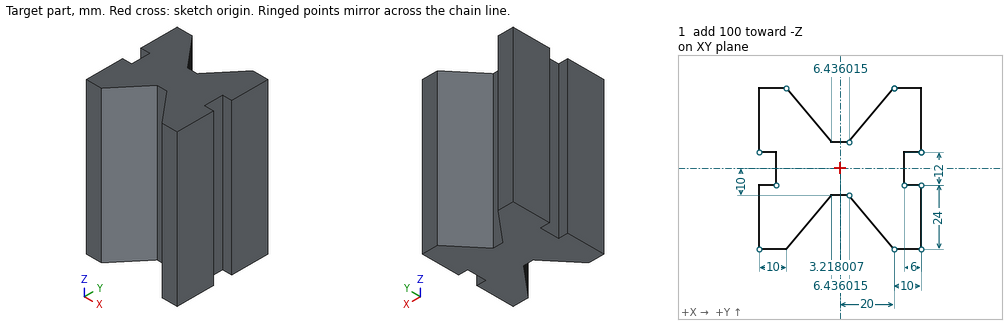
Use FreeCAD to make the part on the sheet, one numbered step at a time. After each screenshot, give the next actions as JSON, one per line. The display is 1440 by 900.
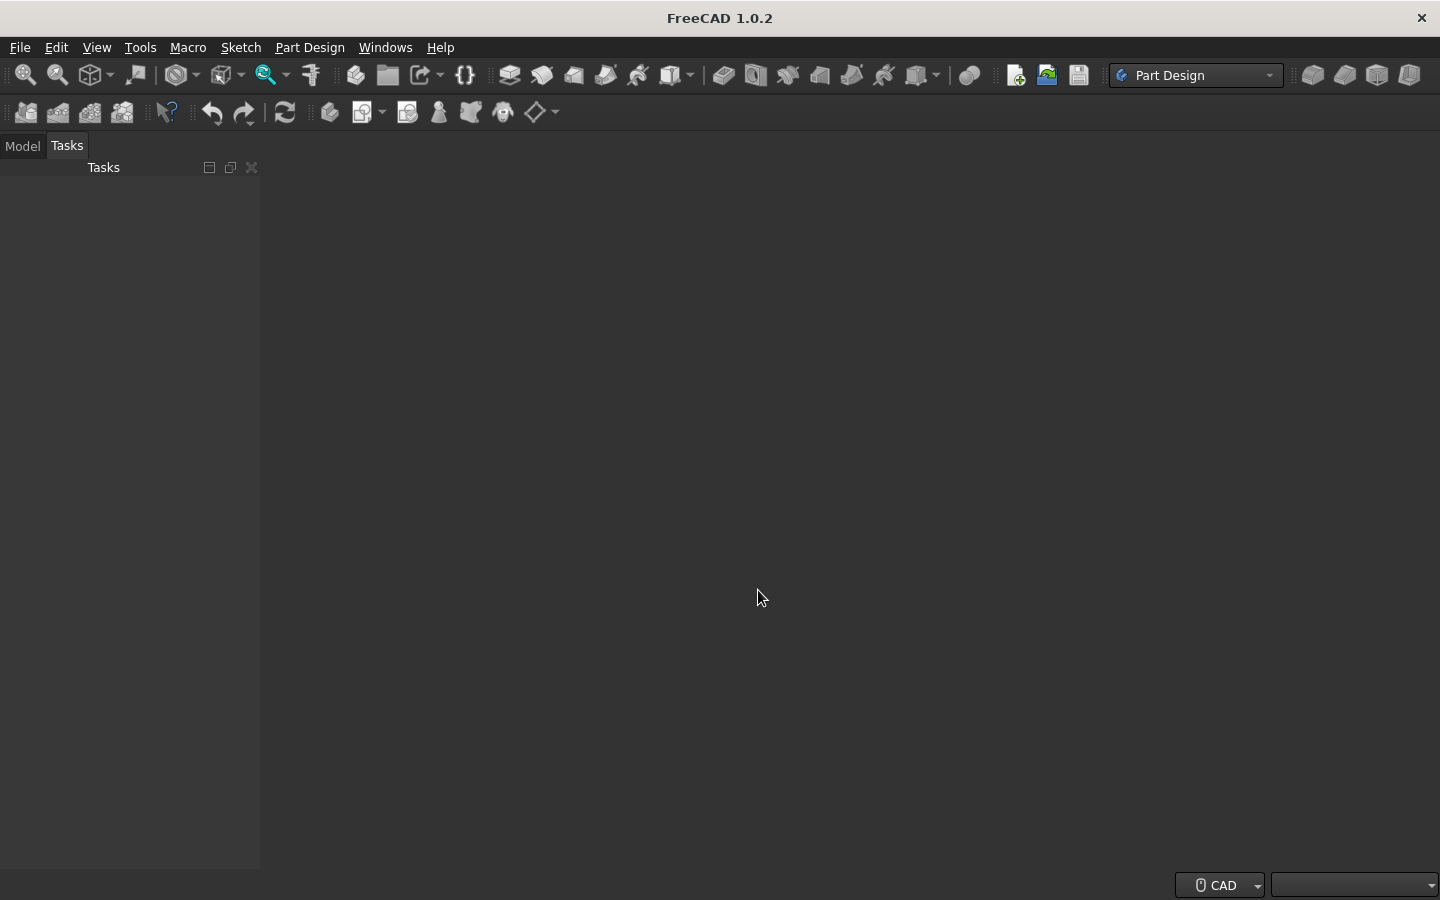
{"action": "key", "text": "ctrl+n"}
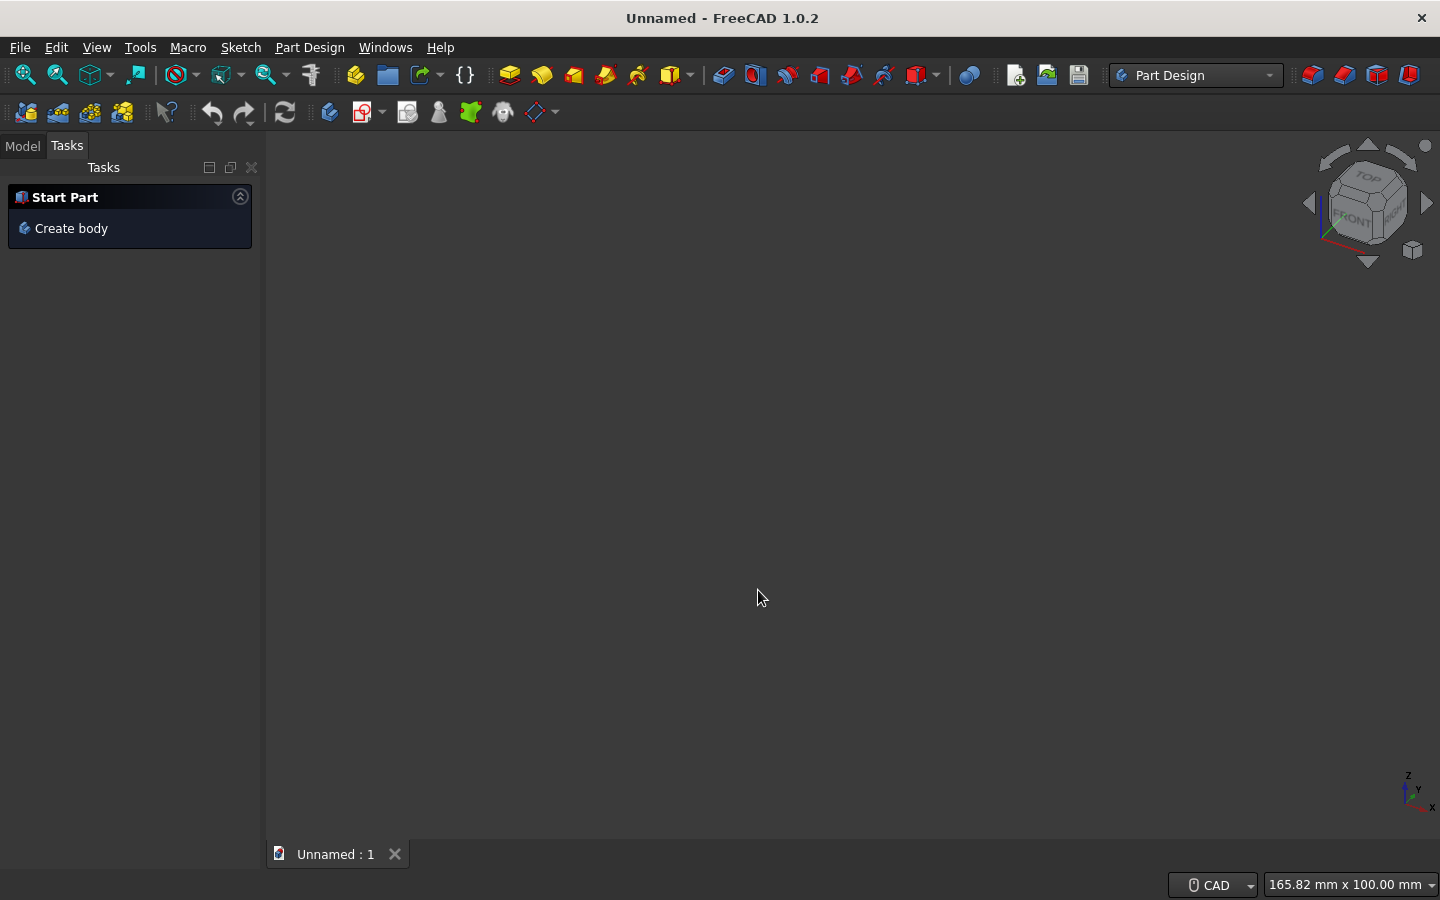
{"action": "left_click", "coordinate": [362, 112]}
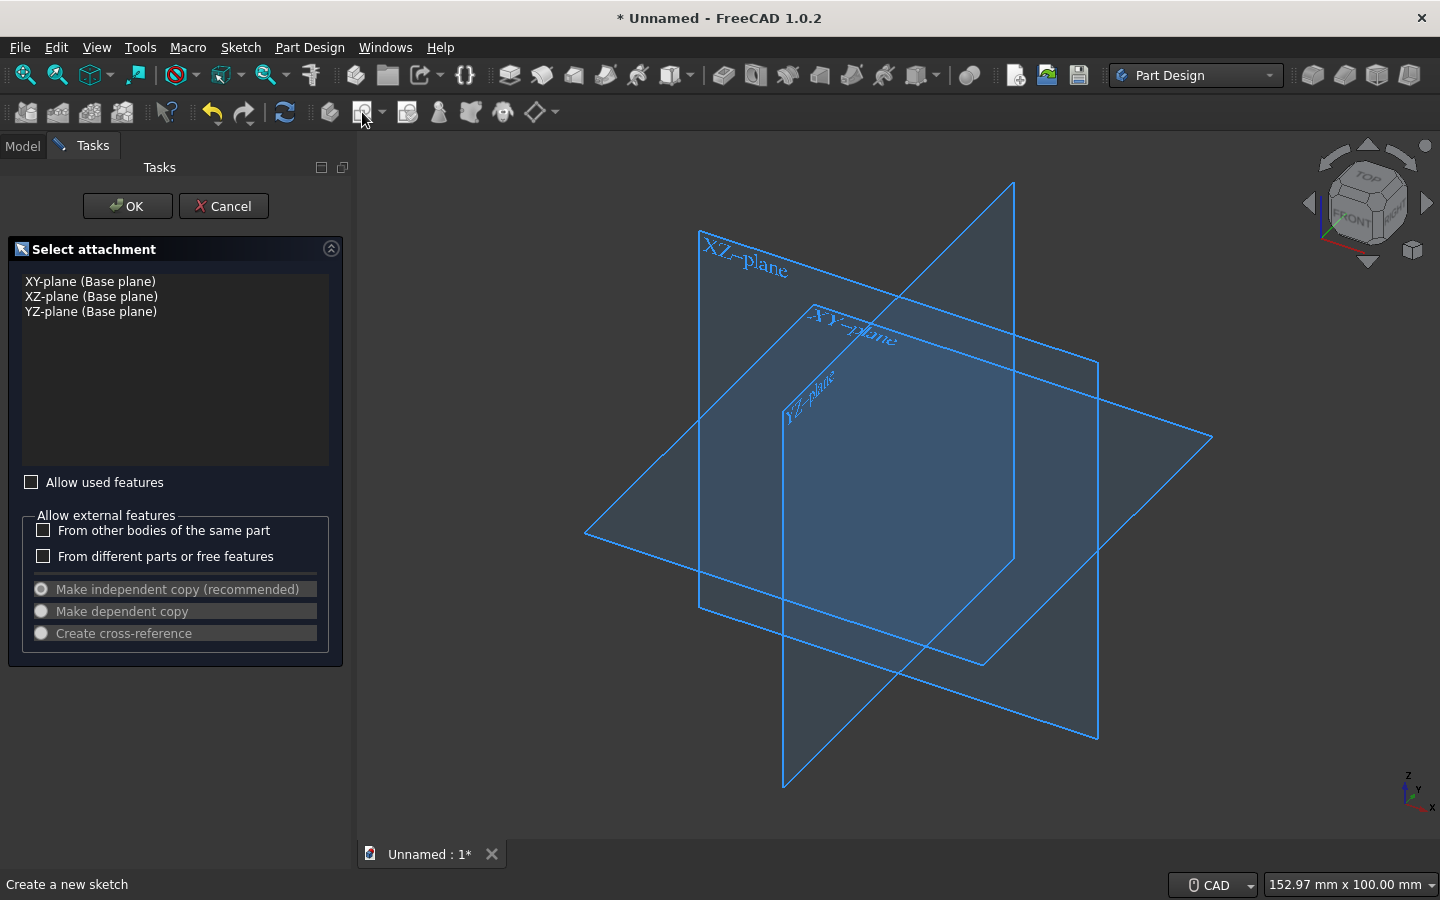
{"action": "left_click", "coordinate": [82, 282]}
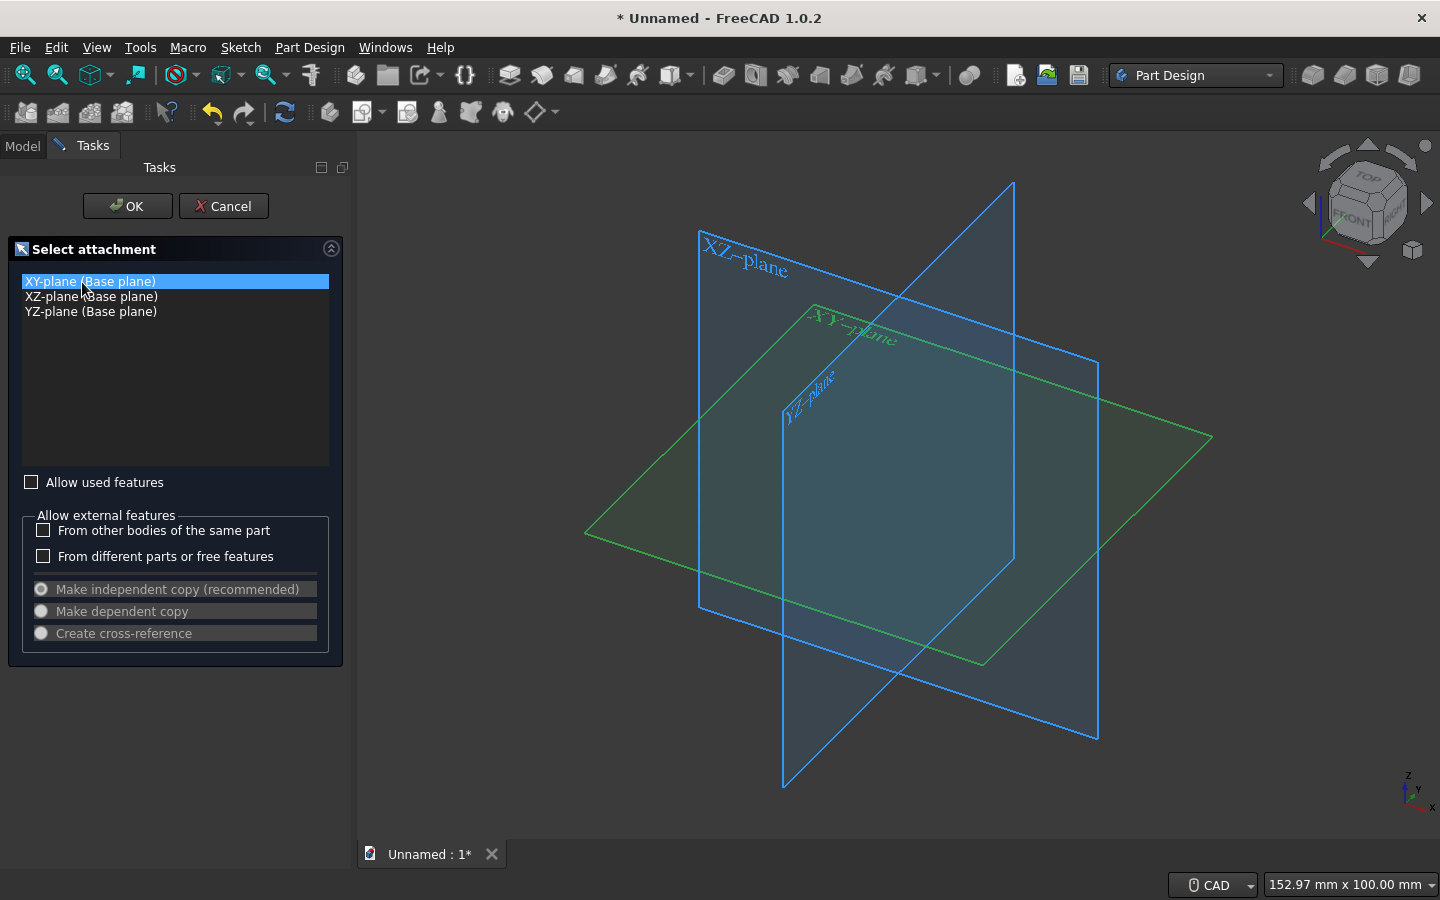
{"action": "left_click", "coordinate": [128, 206]}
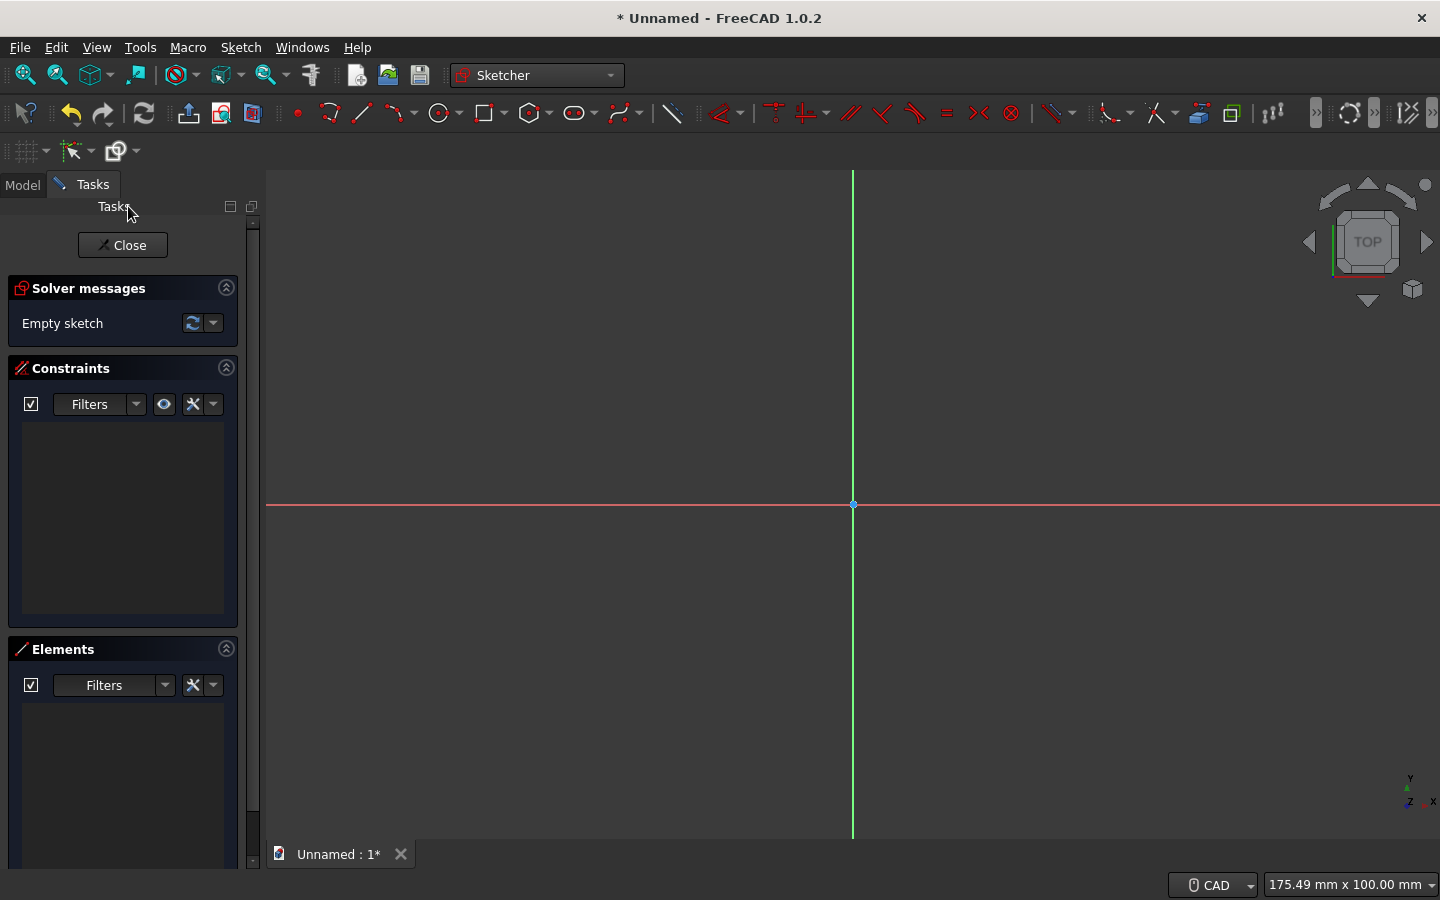
{"action": "key", "text": "g m"}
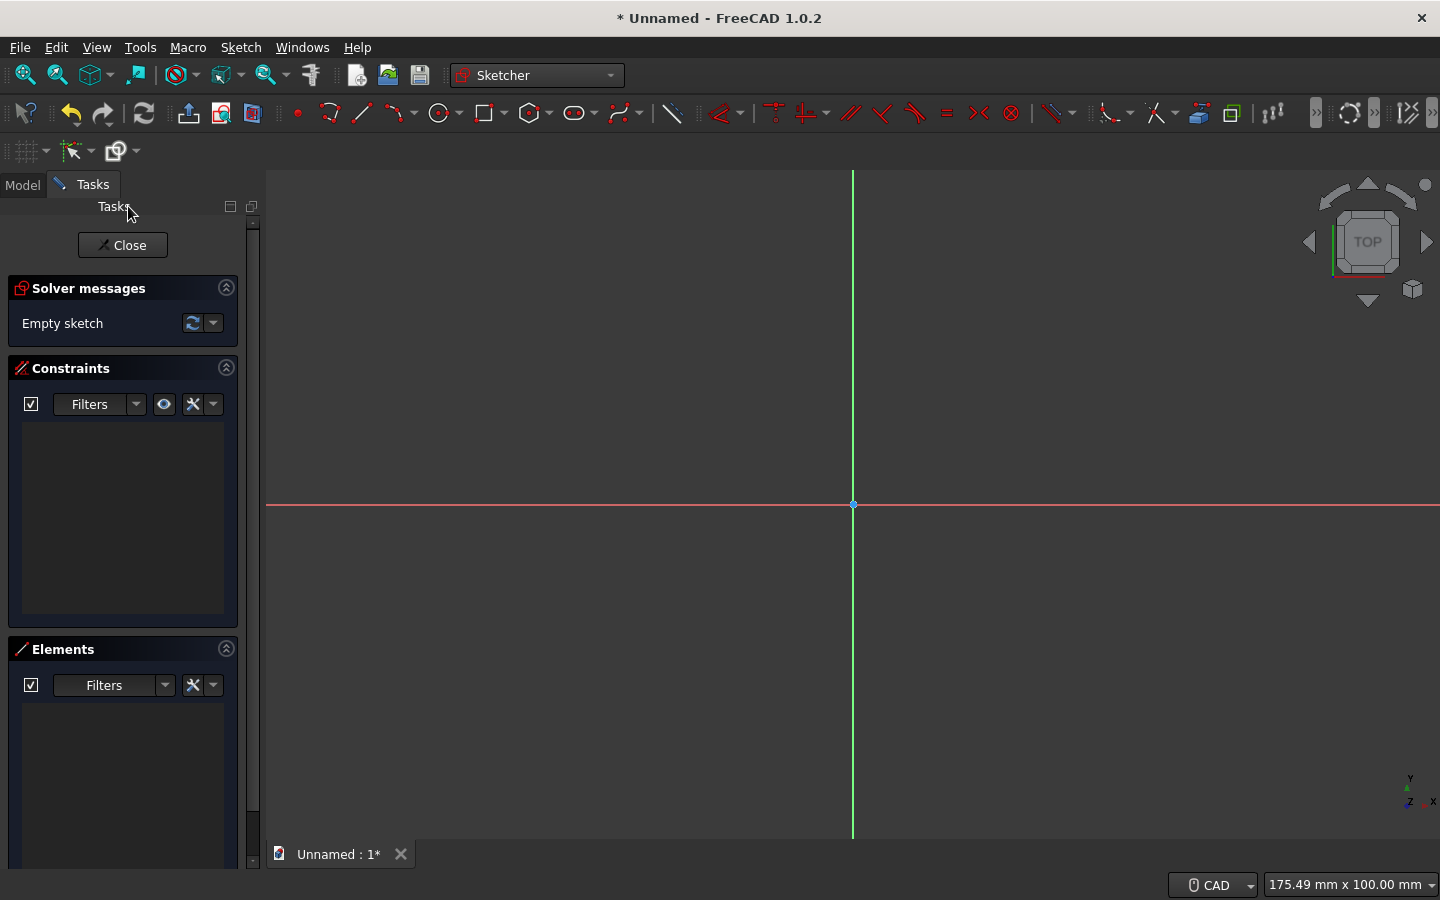
{"action": "left_click", "coordinate": [831, 571]}
{"action": "left_click", "coordinate": [875, 571]}
{"action": "left_click", "coordinate": [987, 705]}
{"action": "left_click", "coordinate": [1054, 705]}
{"action": "left_click", "coordinate": [1054, 545]}
{"action": "left_click", "coordinate": [1014, 545]}
{"action": "left_click", "coordinate": [1014, 464]}
{"action": "left_click", "coordinate": [1054, 464]}
{"action": "left_click", "coordinate": [1054, 304]}
{"action": "left_click", "coordinate": [987, 304]}
{"action": "left_click", "coordinate": [875, 438]}
{"action": "left_click", "coordinate": [831, 438]}
{"action": "left_click", "coordinate": [719, 304]}
{"action": "left_click", "coordinate": [652, 304]}
{"action": "left_click", "coordinate": [652, 464]}
{"action": "left_click", "coordinate": [692, 464]}
{"action": "left_click", "coordinate": [692, 545]}
{"action": "left_click", "coordinate": [652, 545]}
{"action": "left_click", "coordinate": [652, 705]}
{"action": "left_click", "coordinate": [719, 705]}
{"action": "left_click", "coordinate": [831, 572]}
{"action": "key", "text": "Escape"}
{"action": "key", "text": "Escape"}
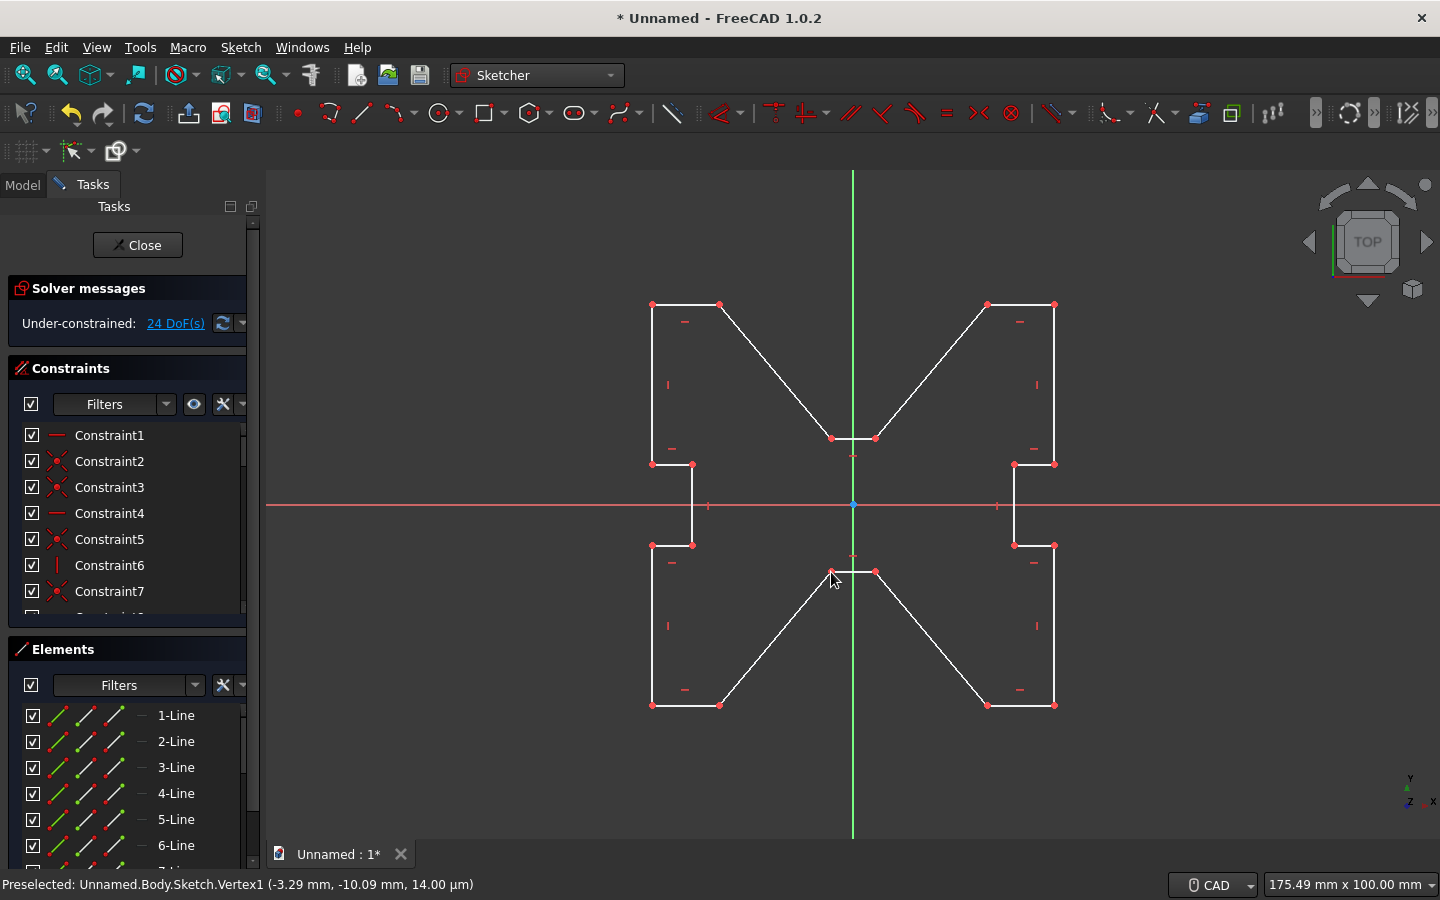
{"action": "left_click", "coordinate": [1054, 546]}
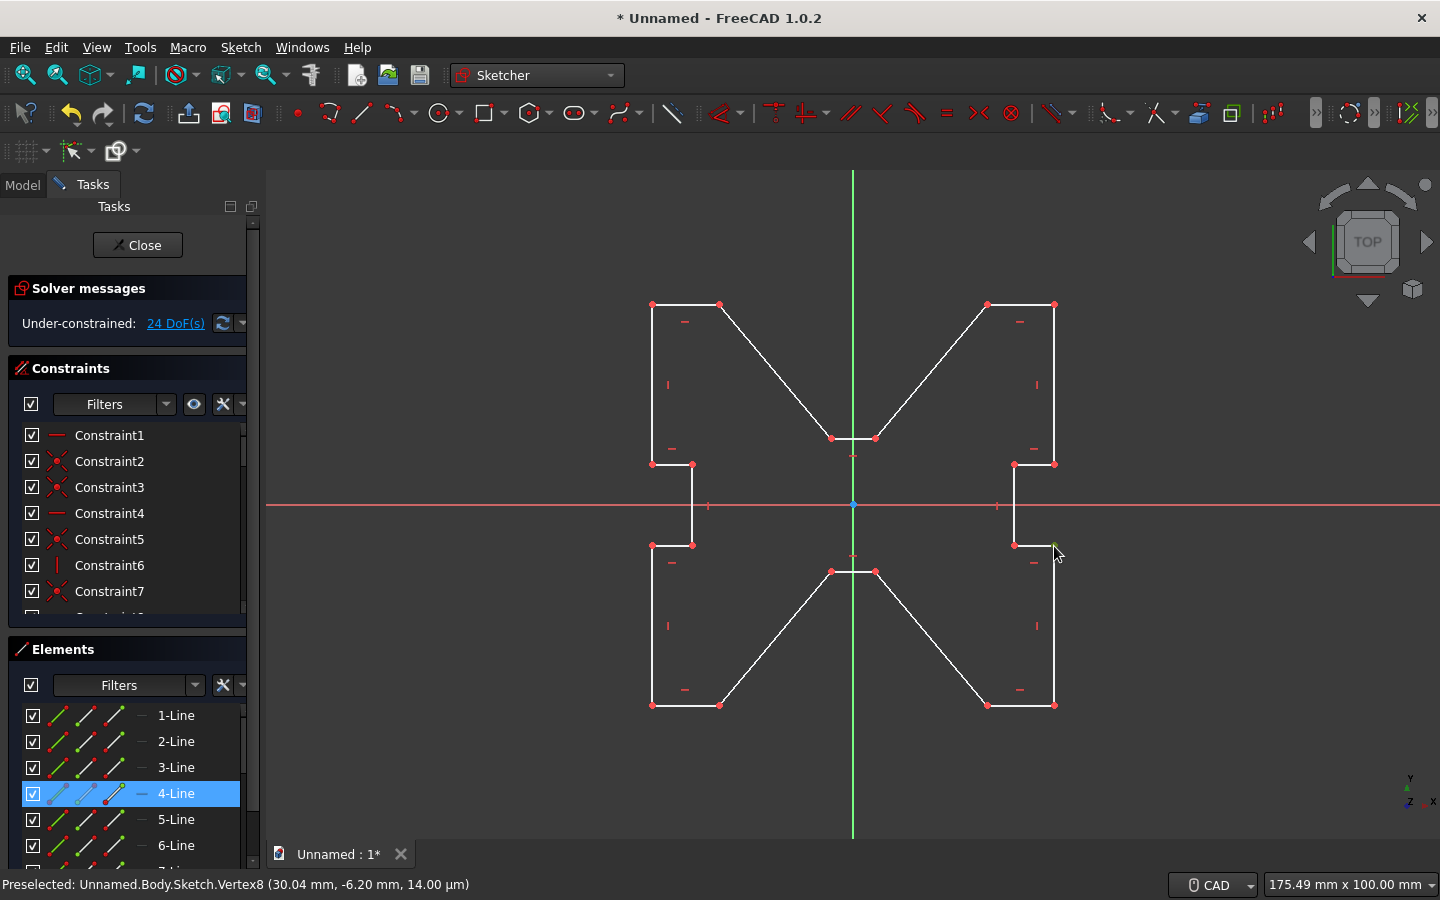
{"action": "left_click", "coordinate": [1054, 465]}